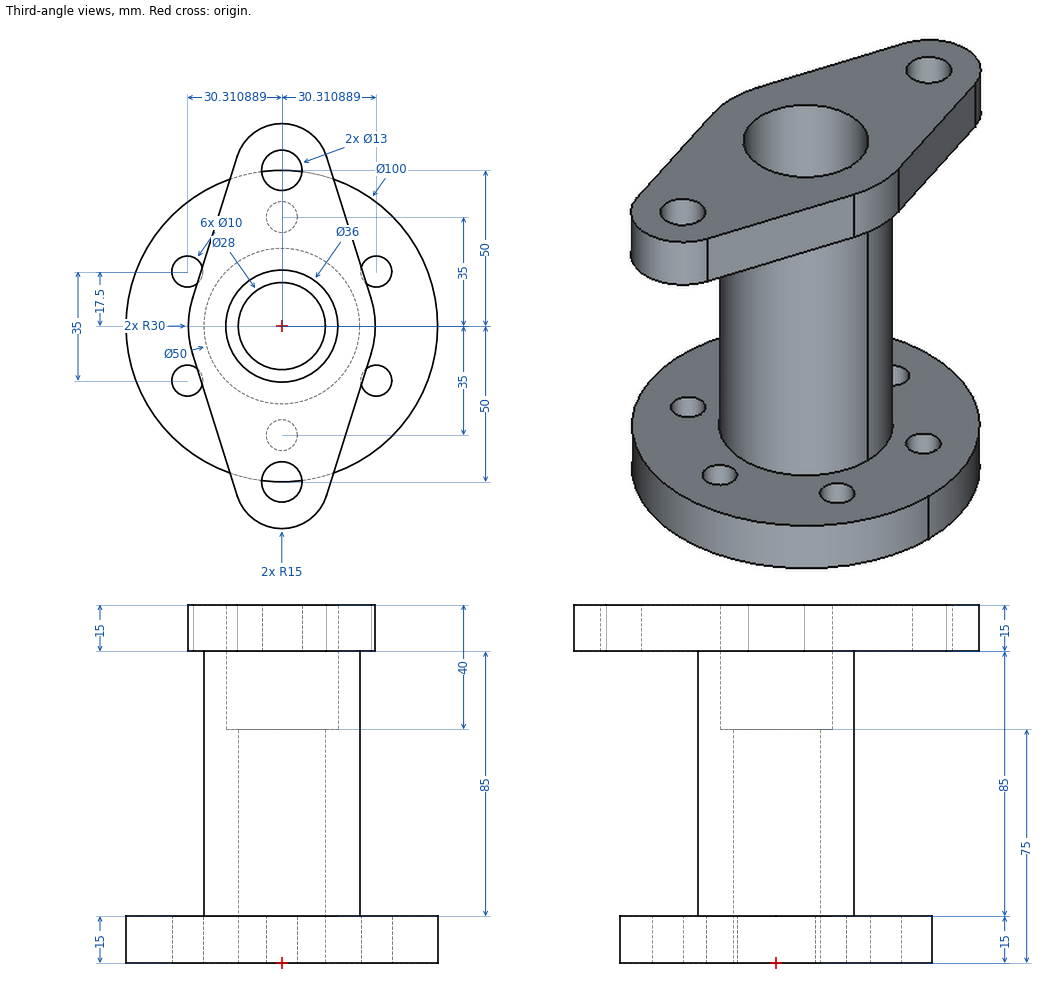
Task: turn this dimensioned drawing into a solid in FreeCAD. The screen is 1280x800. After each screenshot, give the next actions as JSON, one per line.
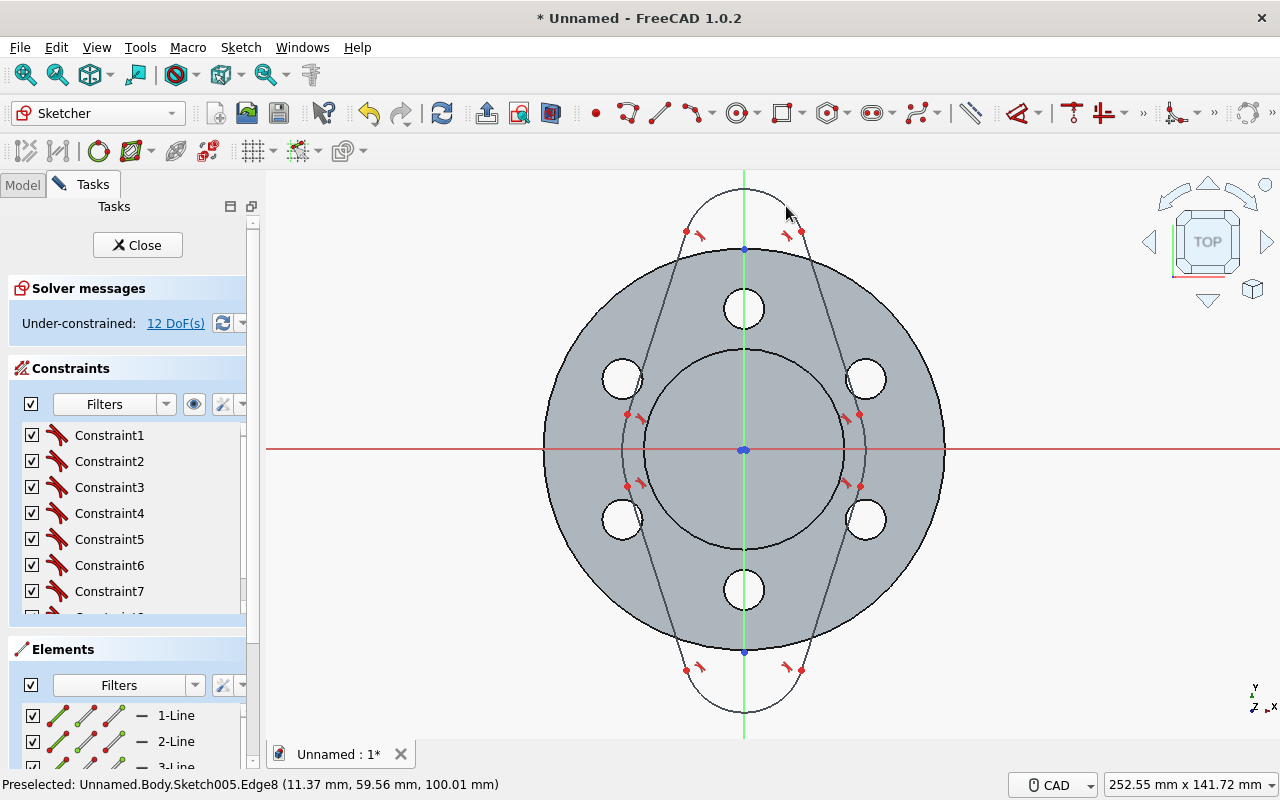
{"action": "left_click", "coordinate": [623, 436]}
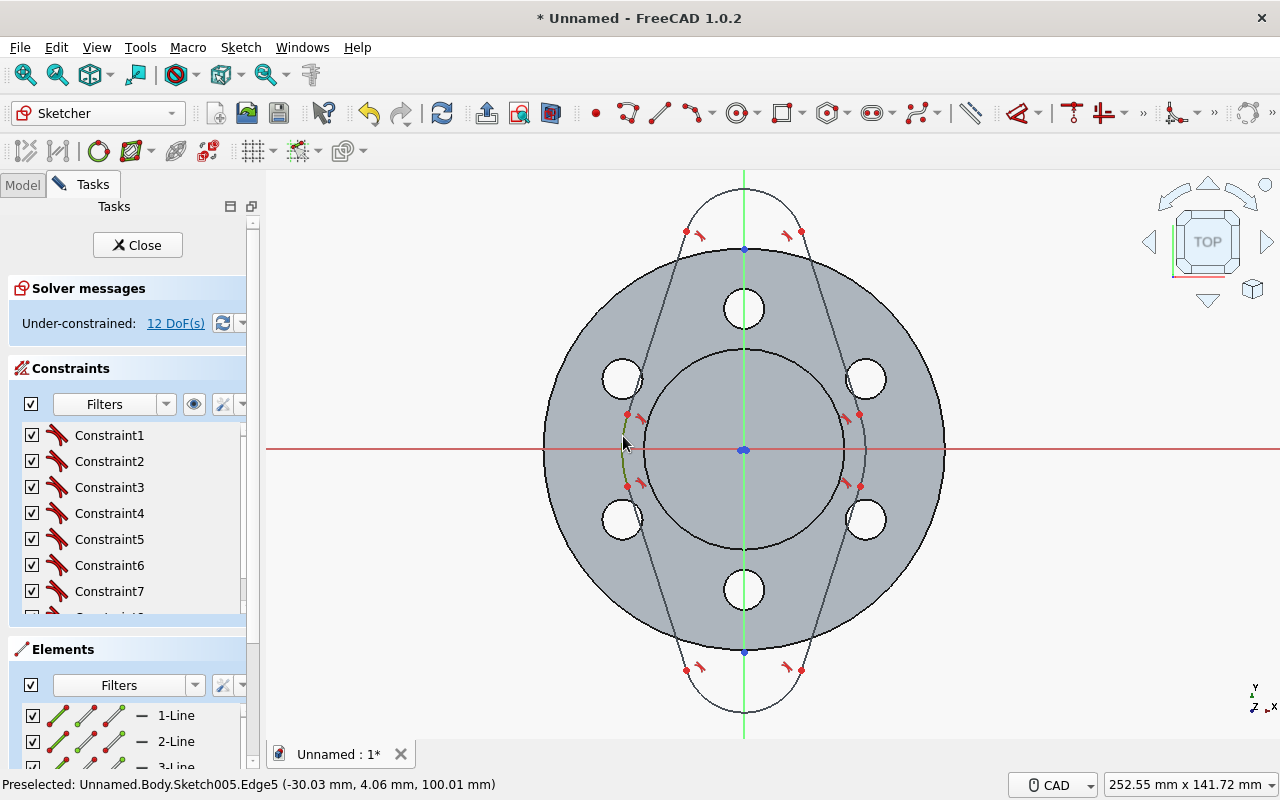
{"action": "left_click", "coordinate": [865, 465]}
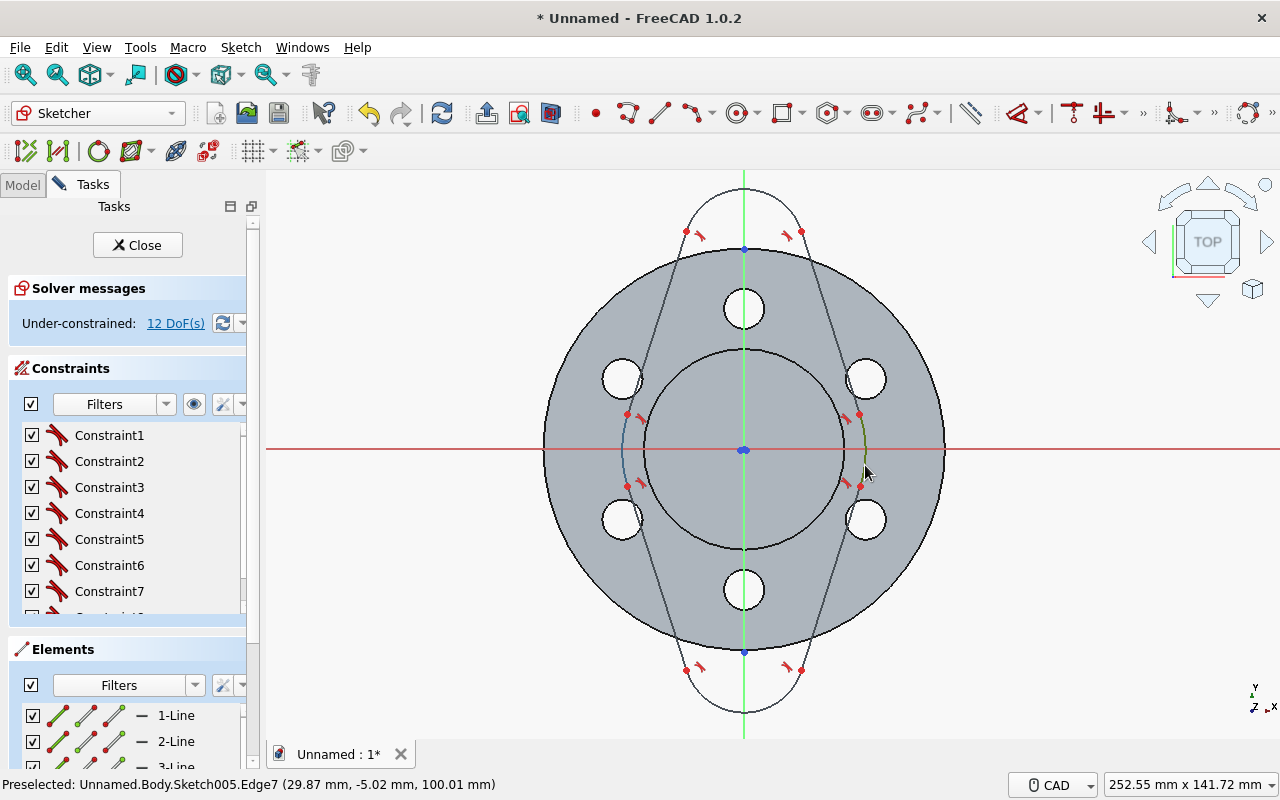
{"action": "key", "text": "c"}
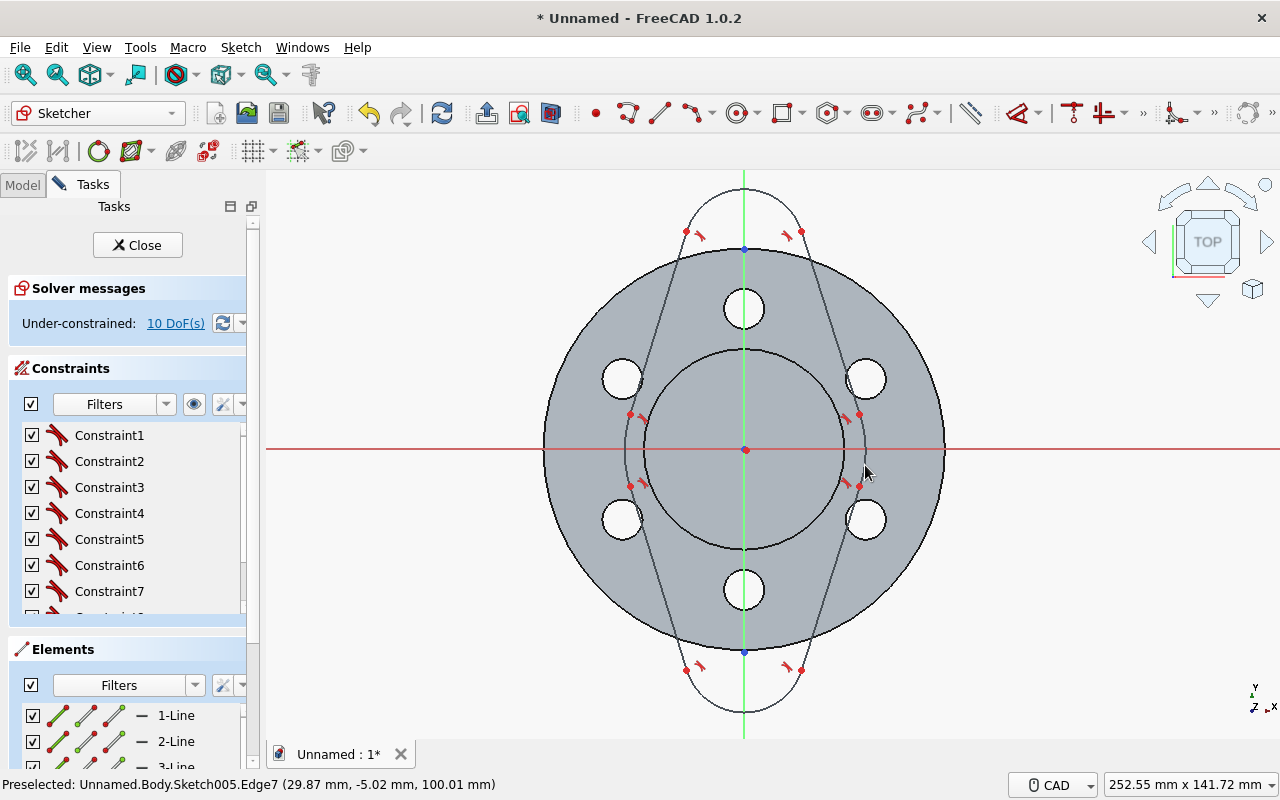
{"action": "left_click_drag", "start_coordinate": [734, 439], "coordinate": [757, 461]}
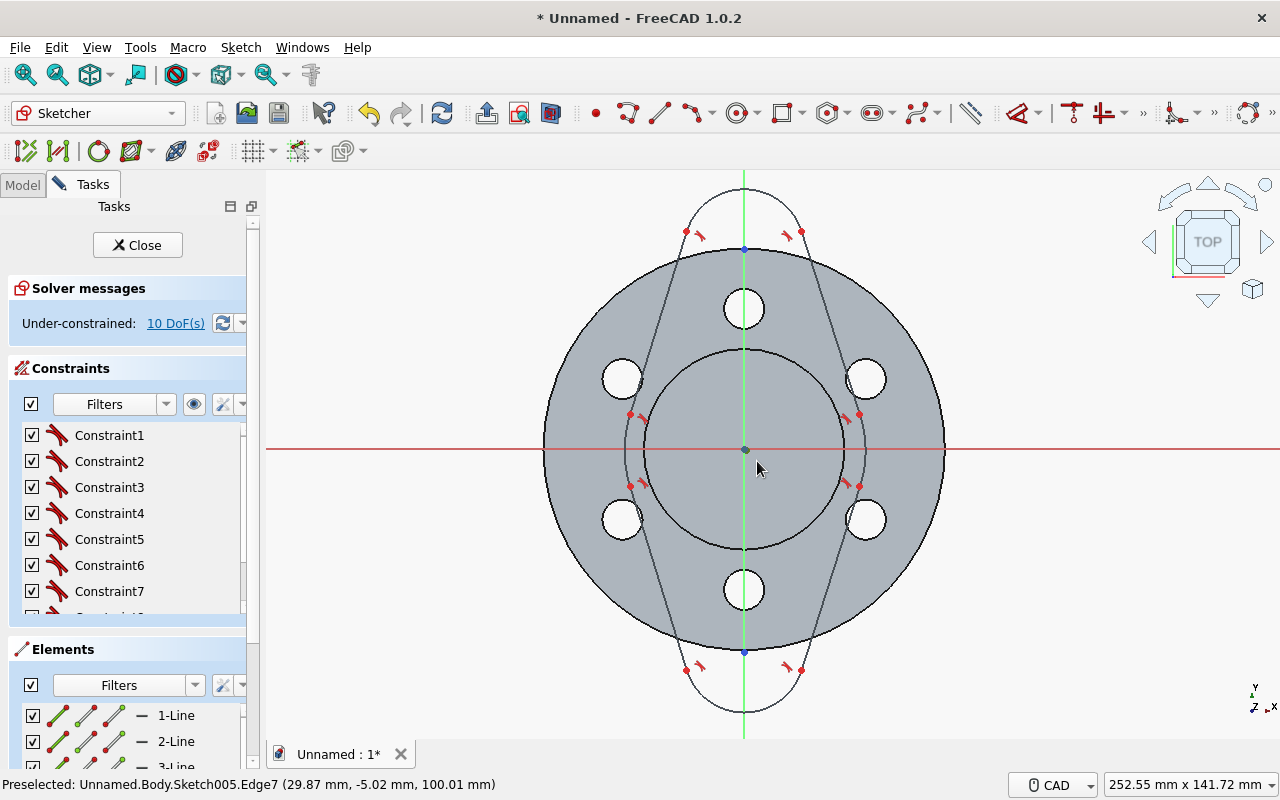
{"action": "left_click", "coordinate": [1072, 114]}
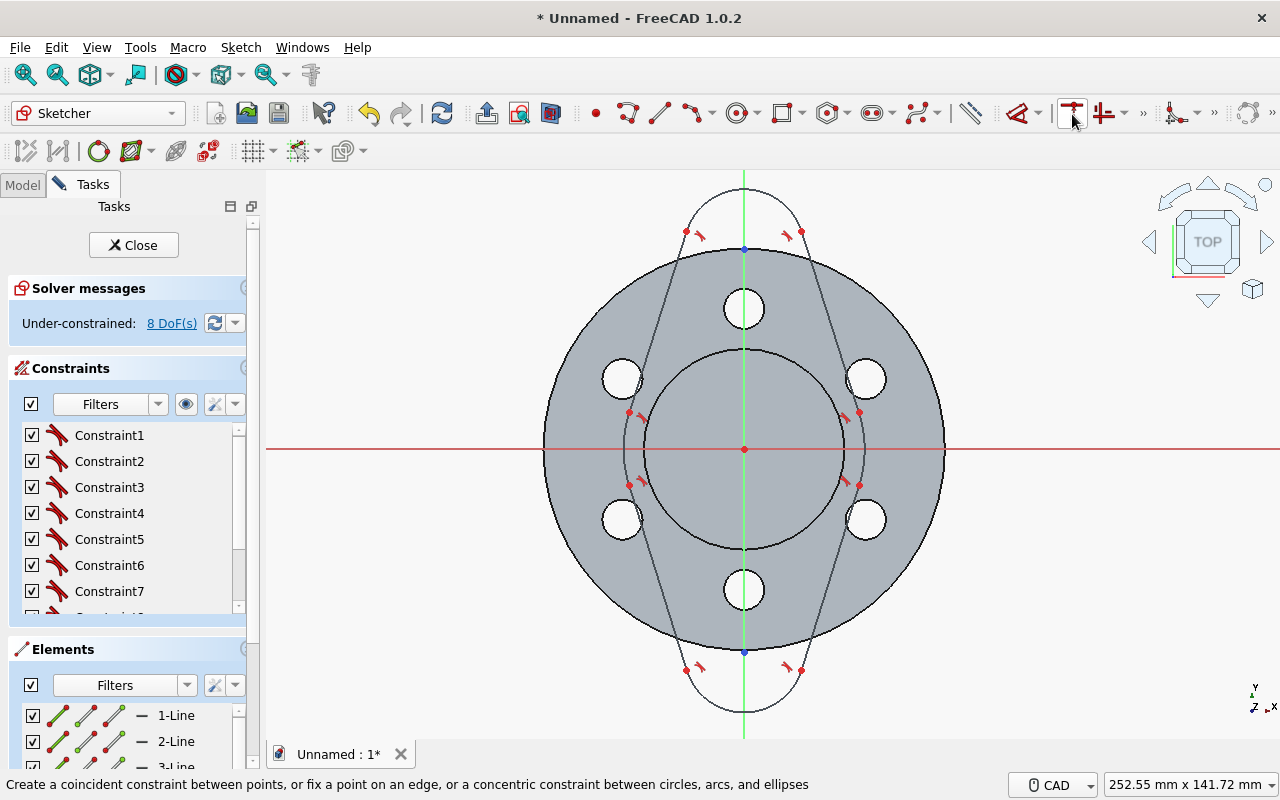
{"action": "left_click", "coordinate": [625, 434]}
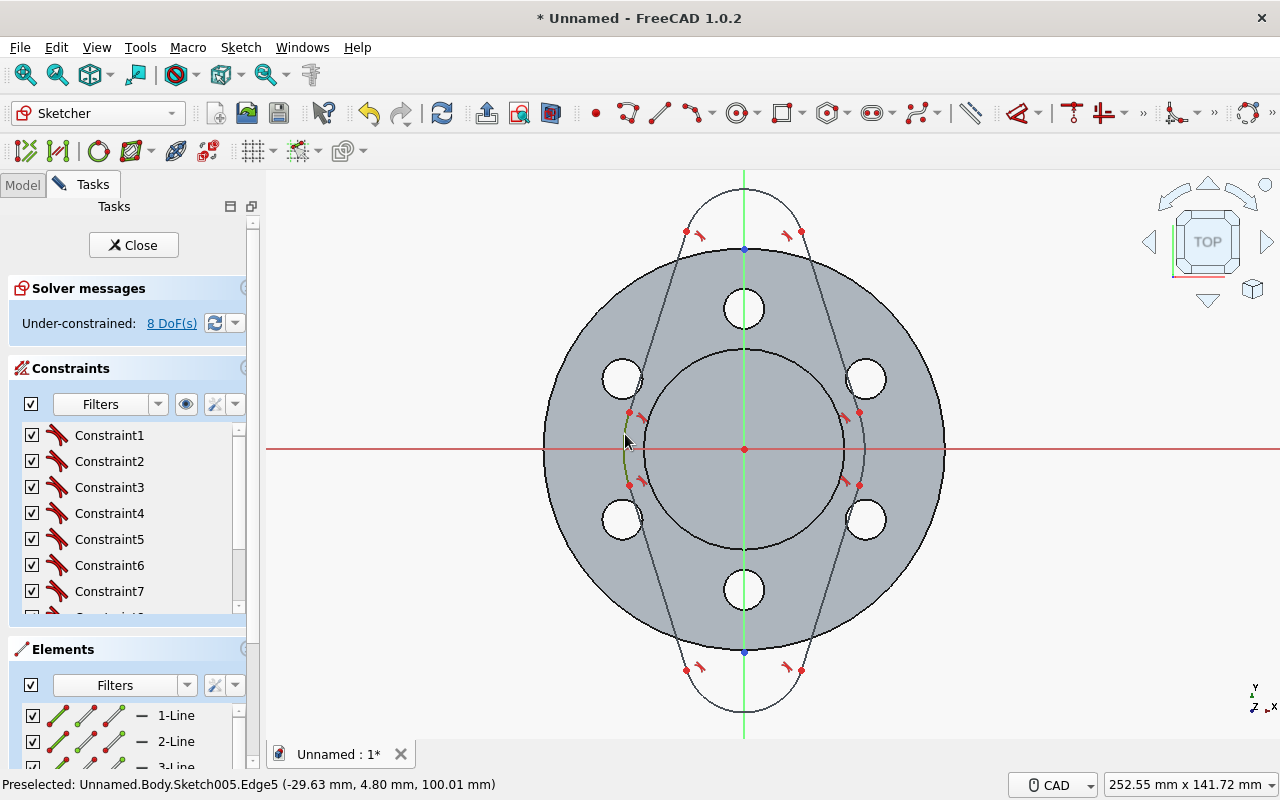
{"action": "left_click", "coordinate": [864, 464]}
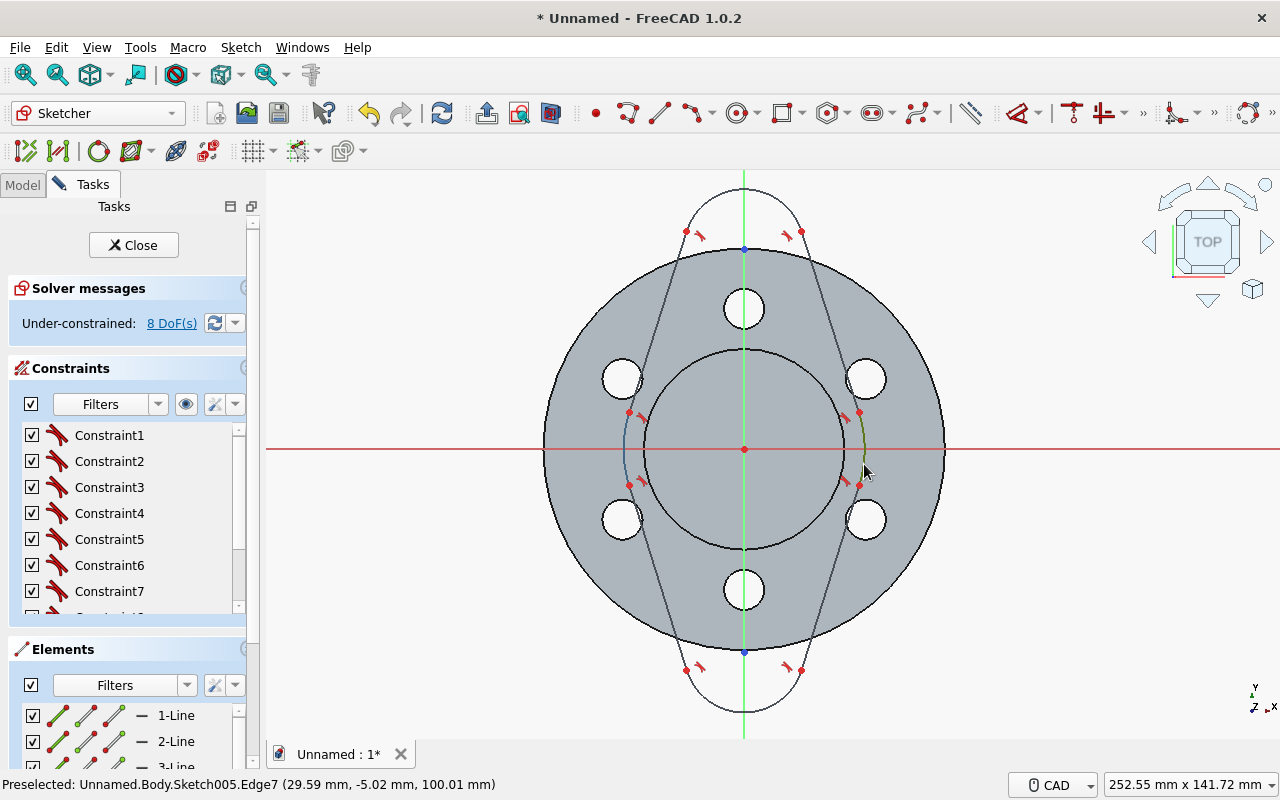
{"action": "key", "text": "e"}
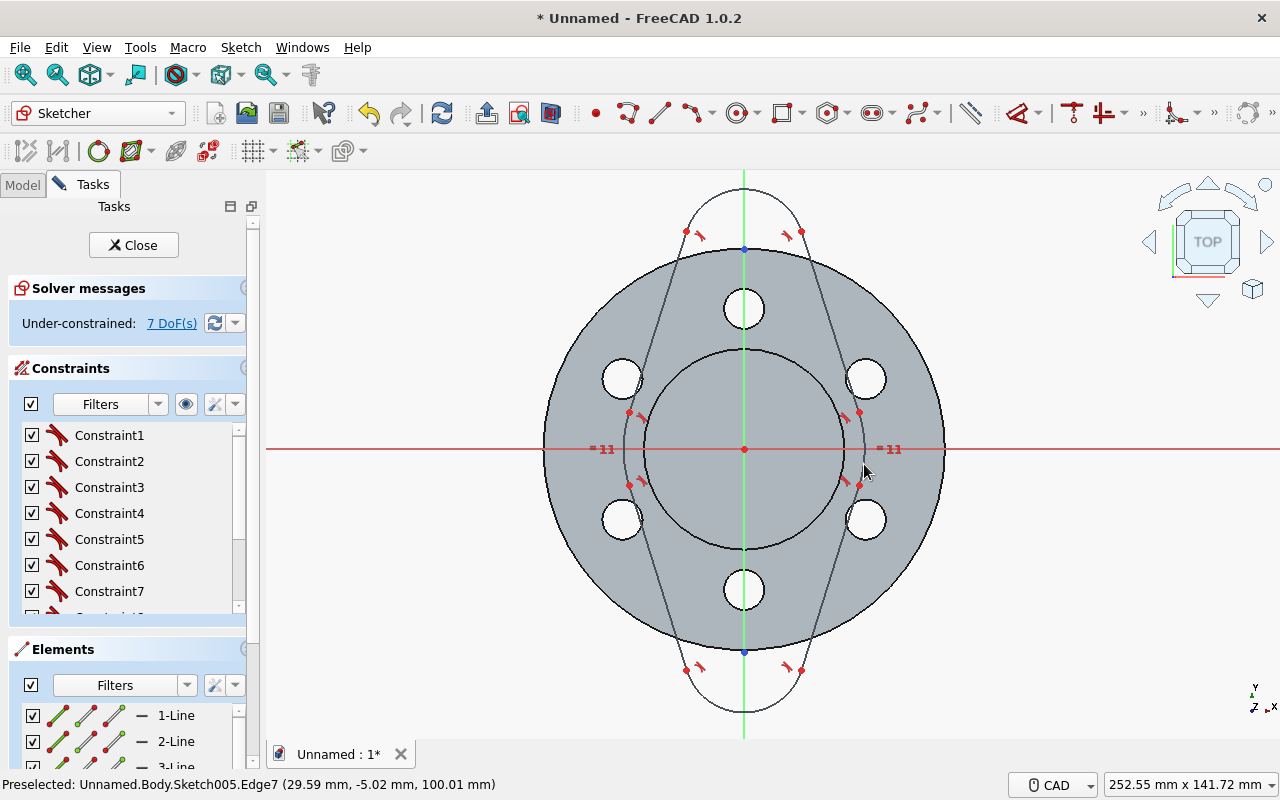
{"action": "left_click", "coordinate": [715, 705]}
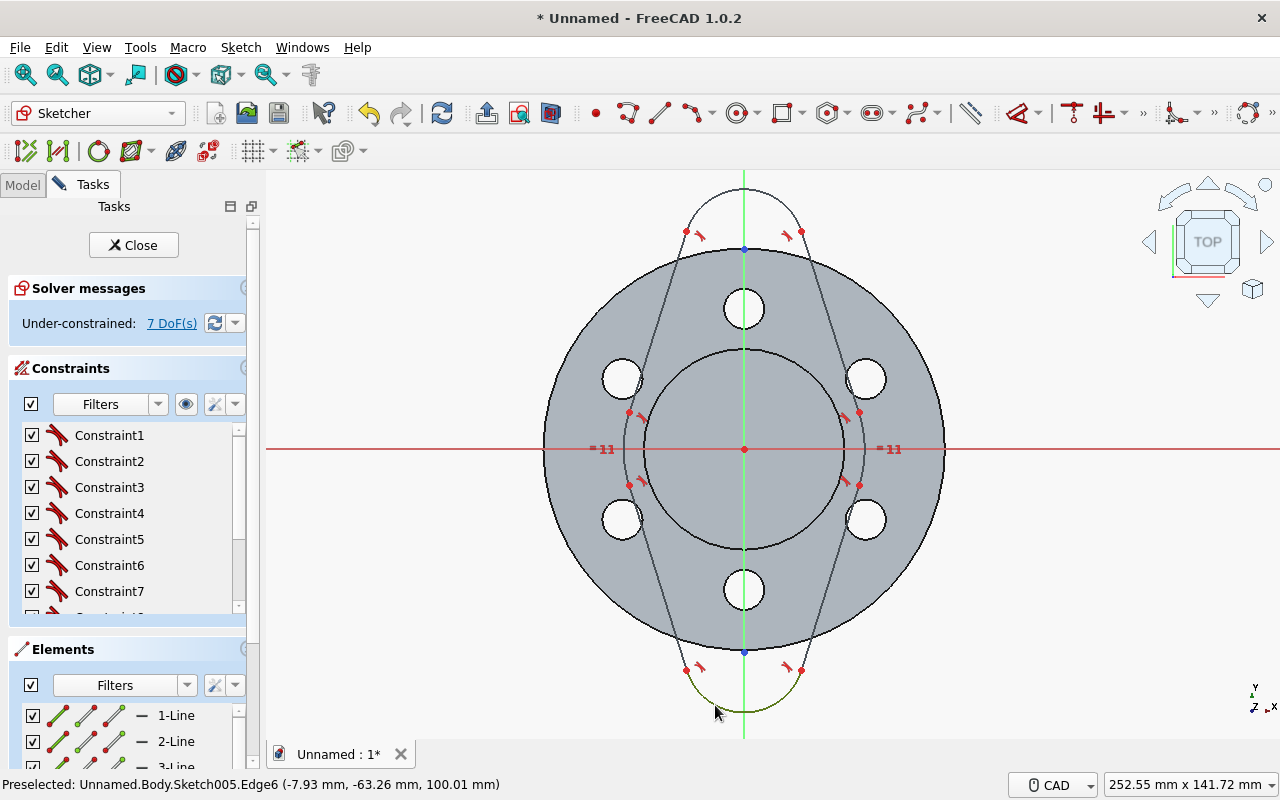
{"action": "left_click", "coordinate": [786, 206]}